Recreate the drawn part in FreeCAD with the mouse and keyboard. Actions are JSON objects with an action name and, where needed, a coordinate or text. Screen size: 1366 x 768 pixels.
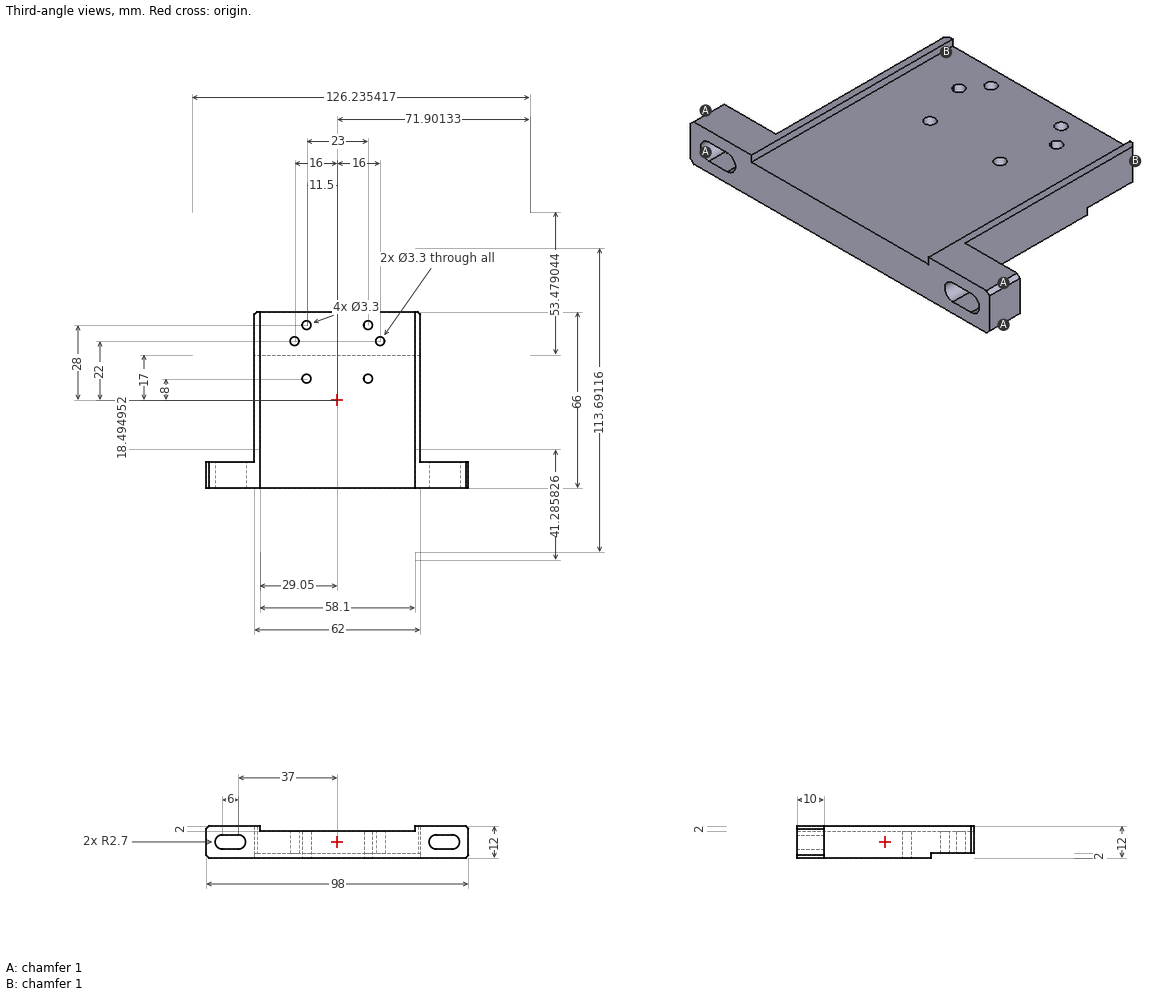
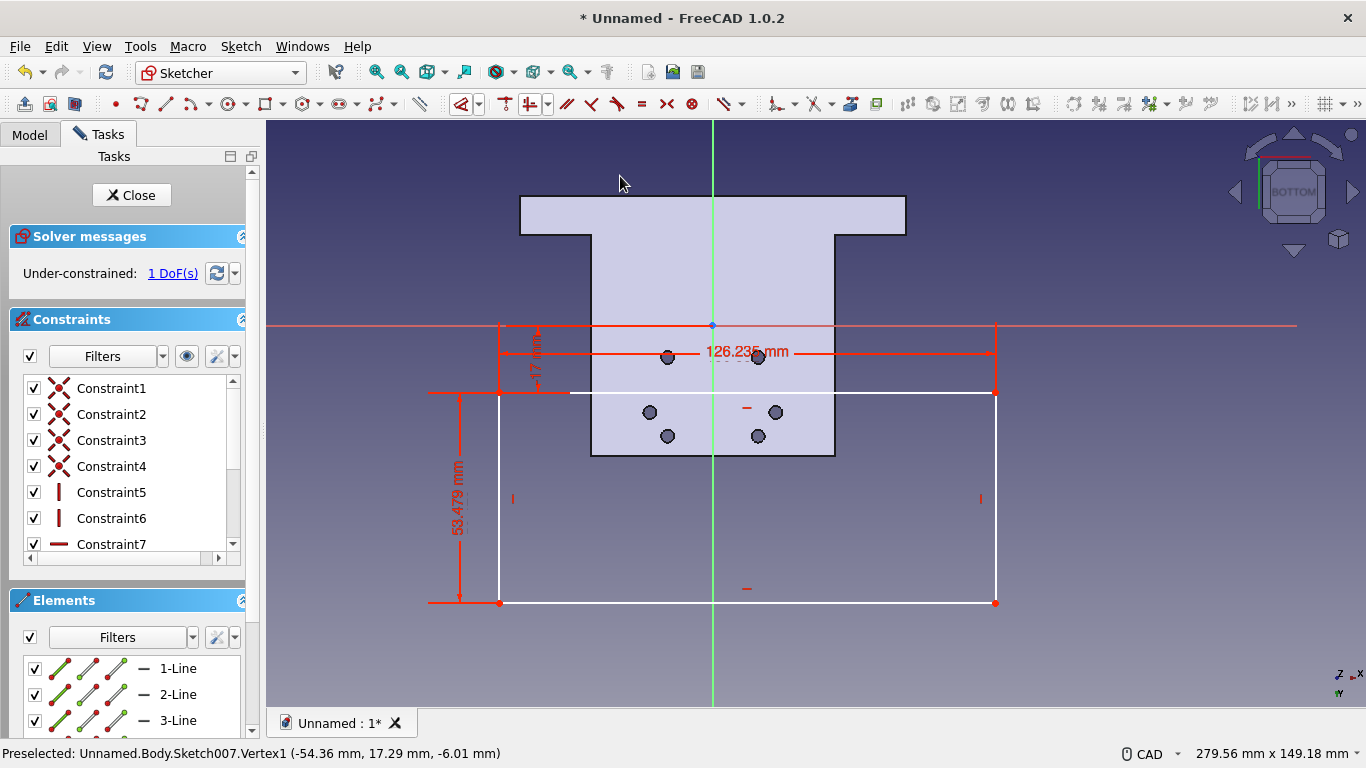
{"action": "left_click", "coordinate": [996, 603]}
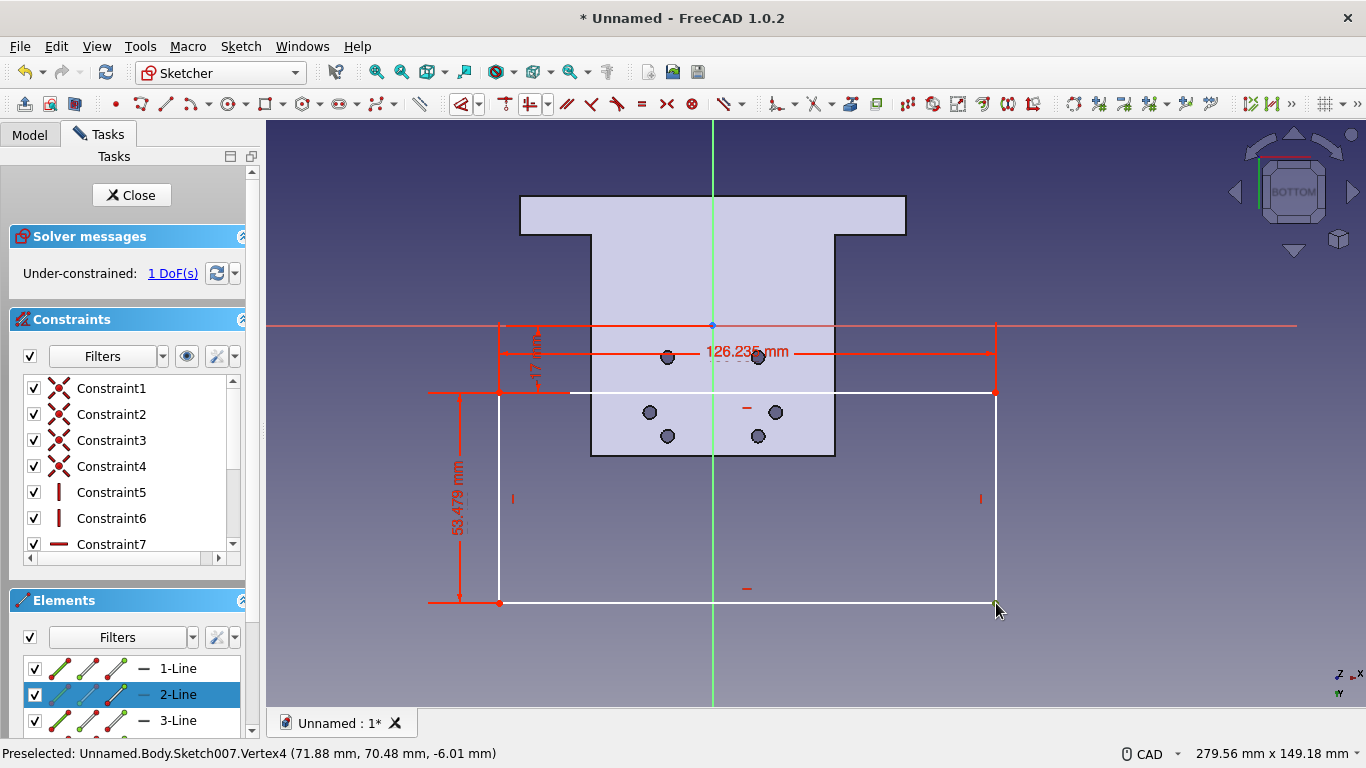
{"action": "left_click", "coordinate": [478, 104]}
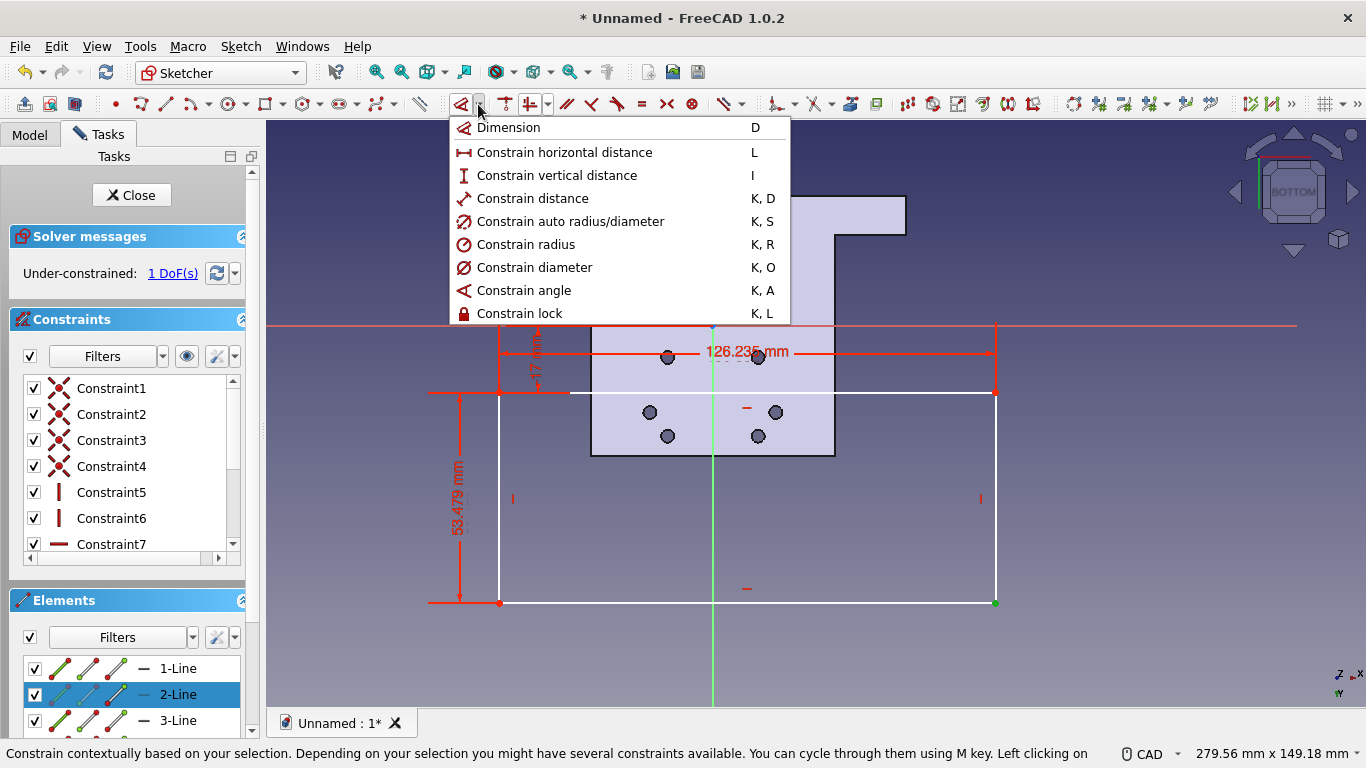
{"action": "left_click", "coordinate": [620, 152]}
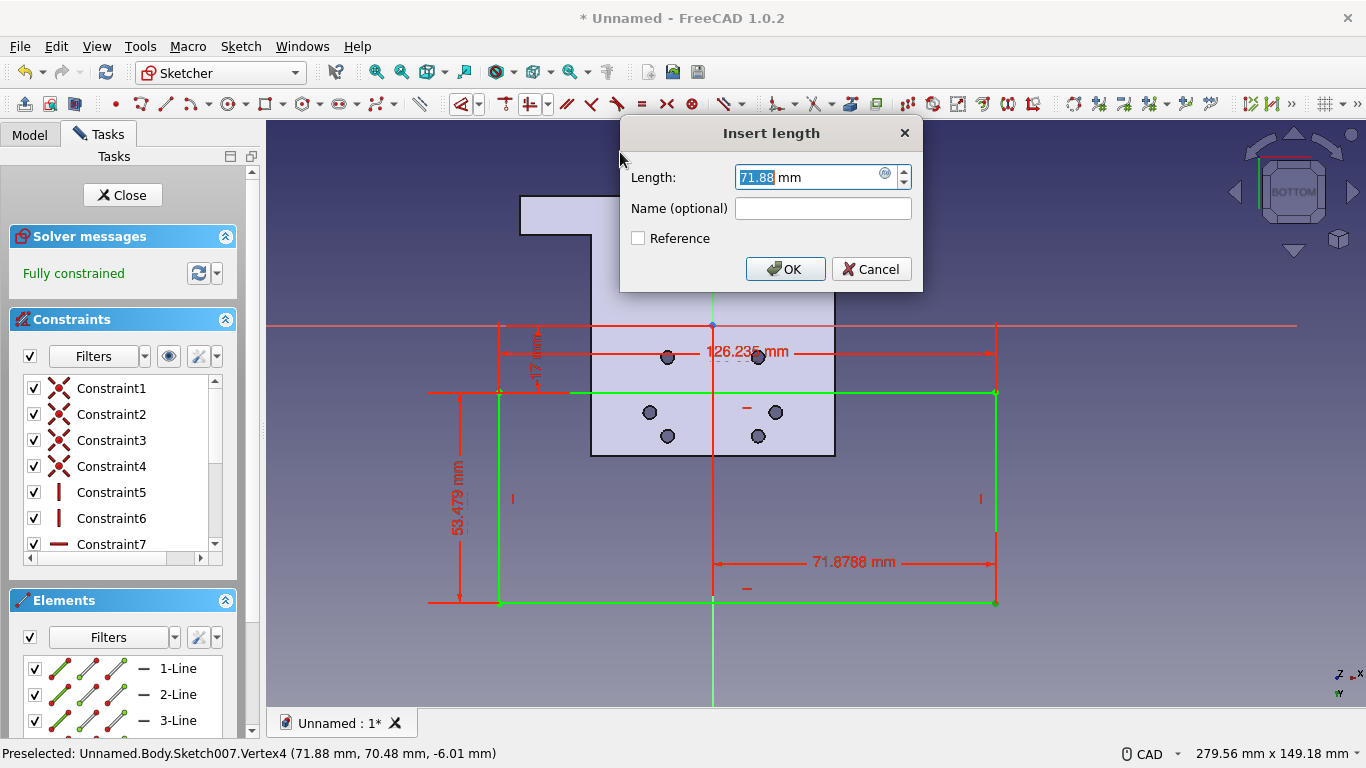
{"action": "type", "text": "71.90133"}
{"action": "key", "text": "Return"}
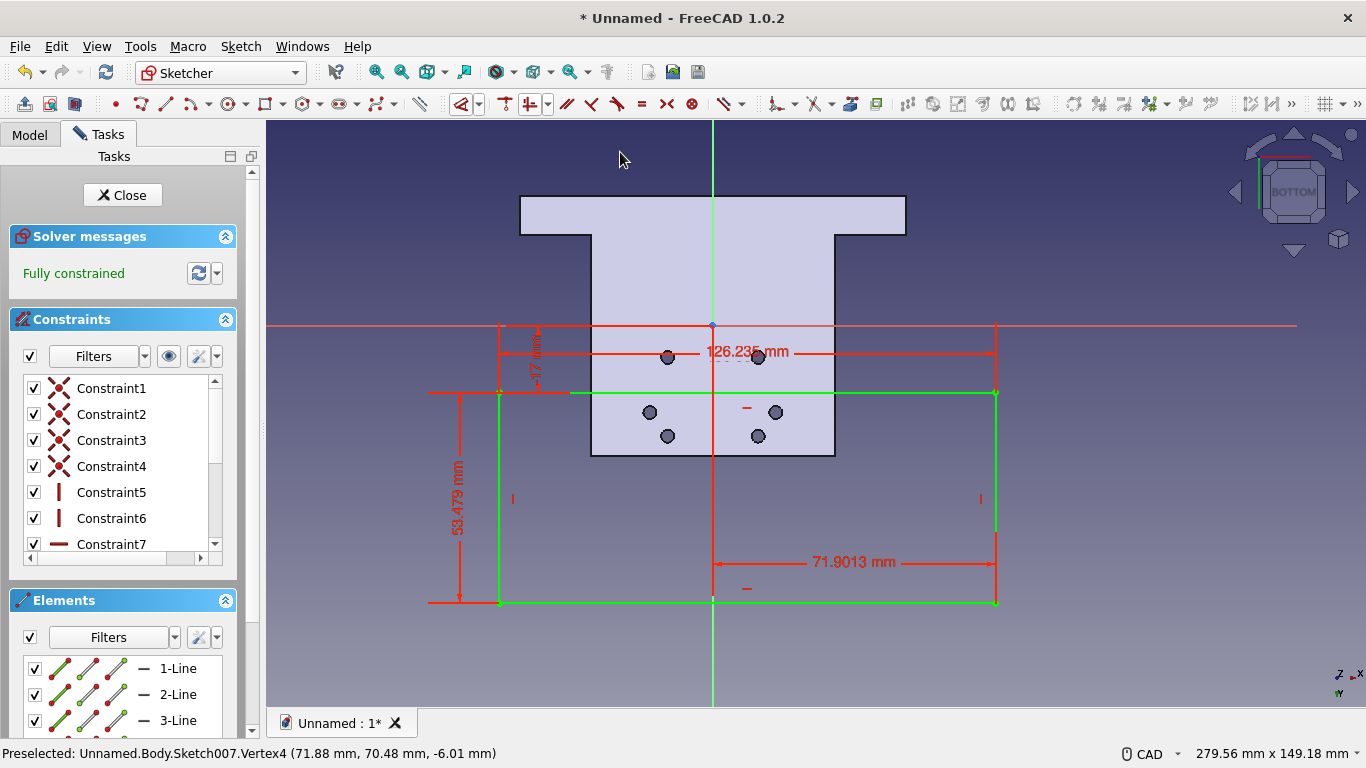
{"action": "left_click", "coordinate": [123, 195]}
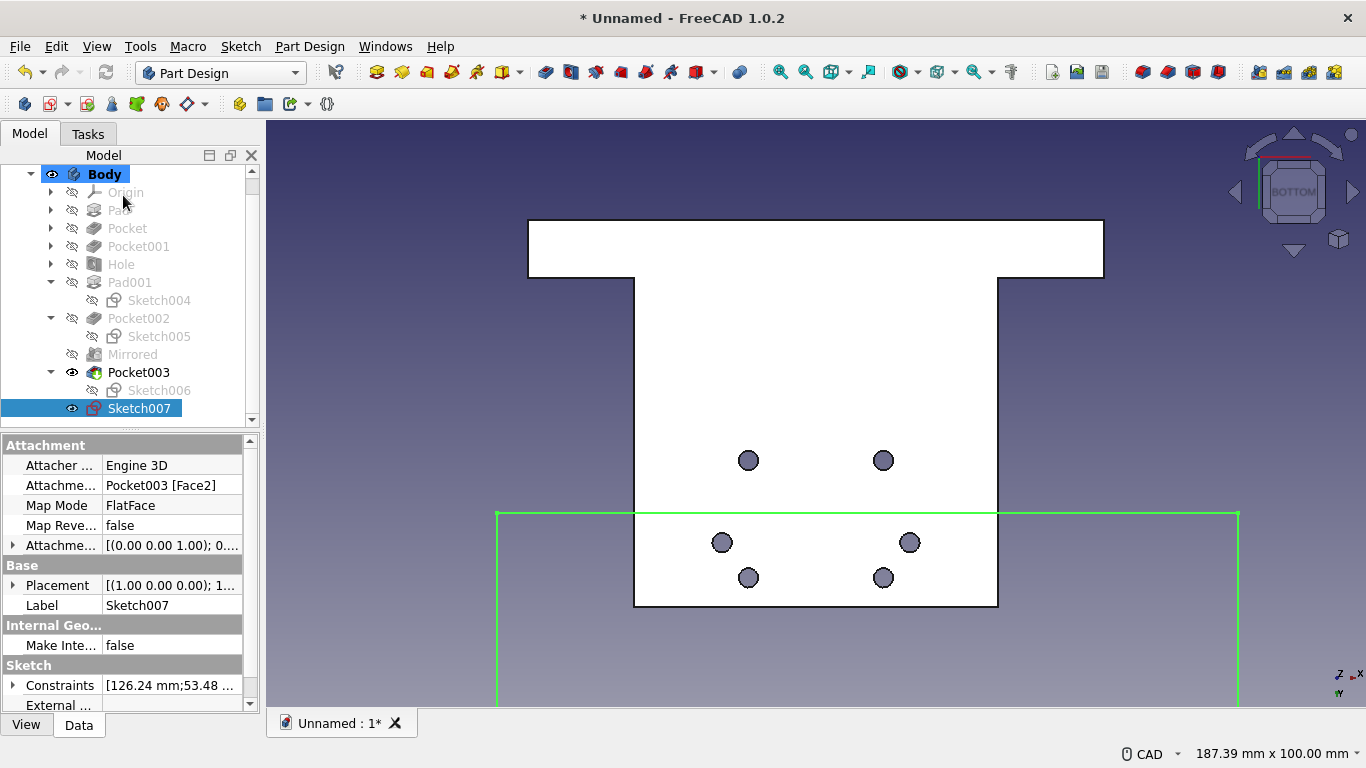
{"action": "left_click", "coordinate": [546, 72]}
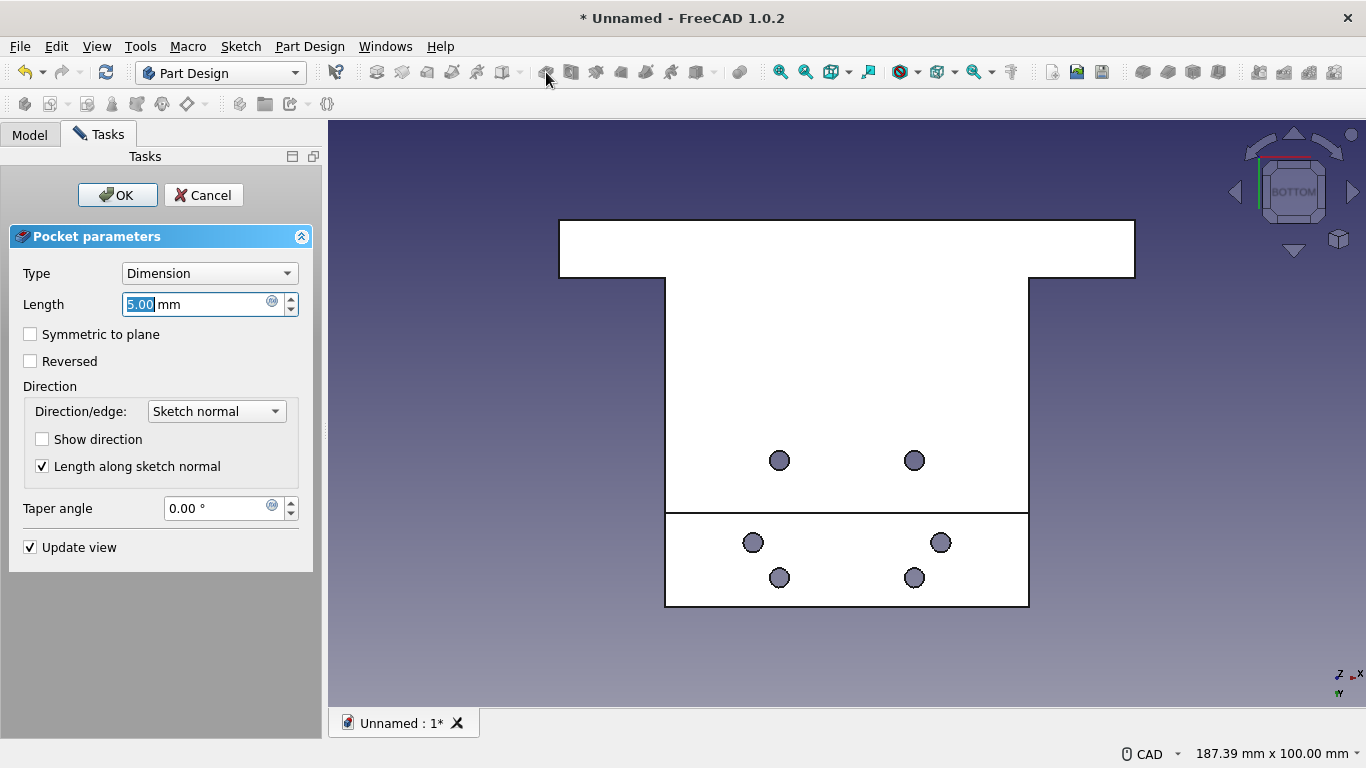
{"action": "type", "text": "2"}
{"action": "key", "text": "Tab"}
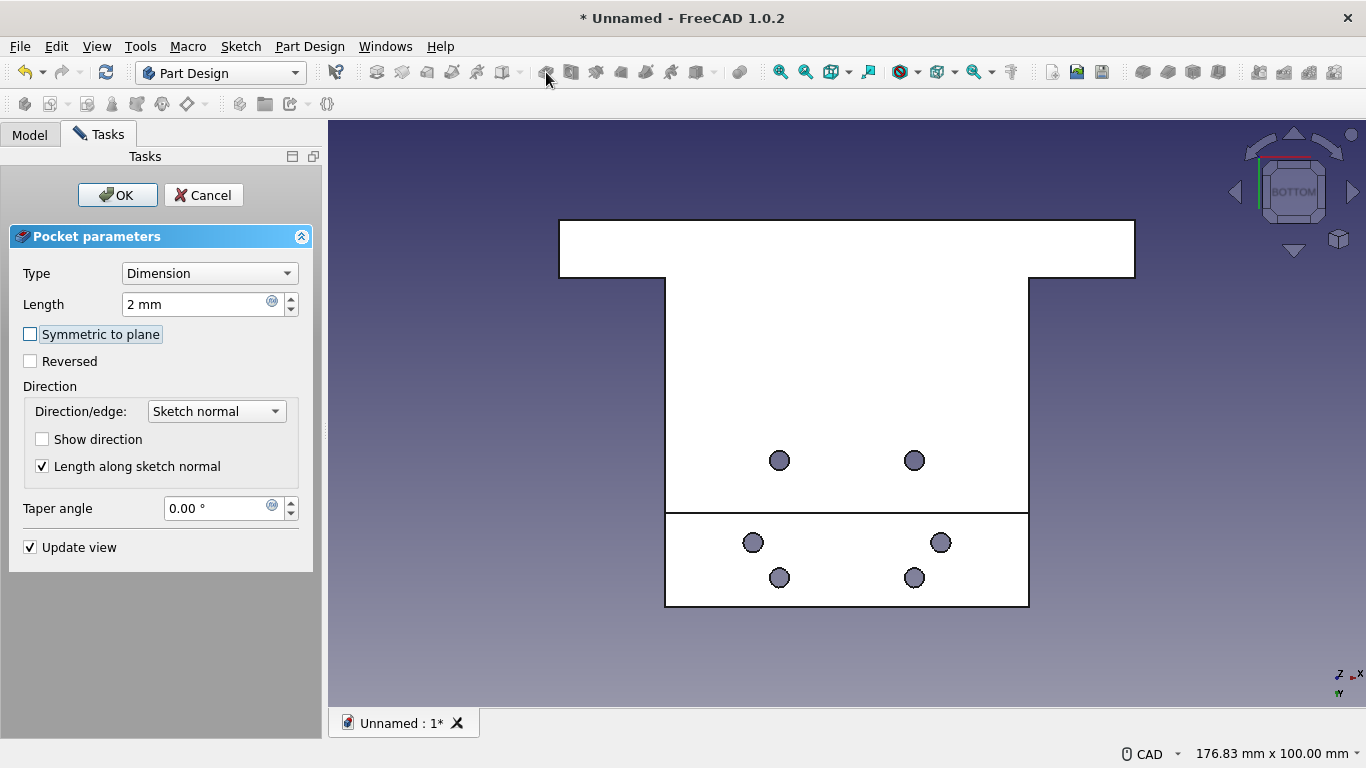
{"action": "left_click", "coordinate": [118, 195]}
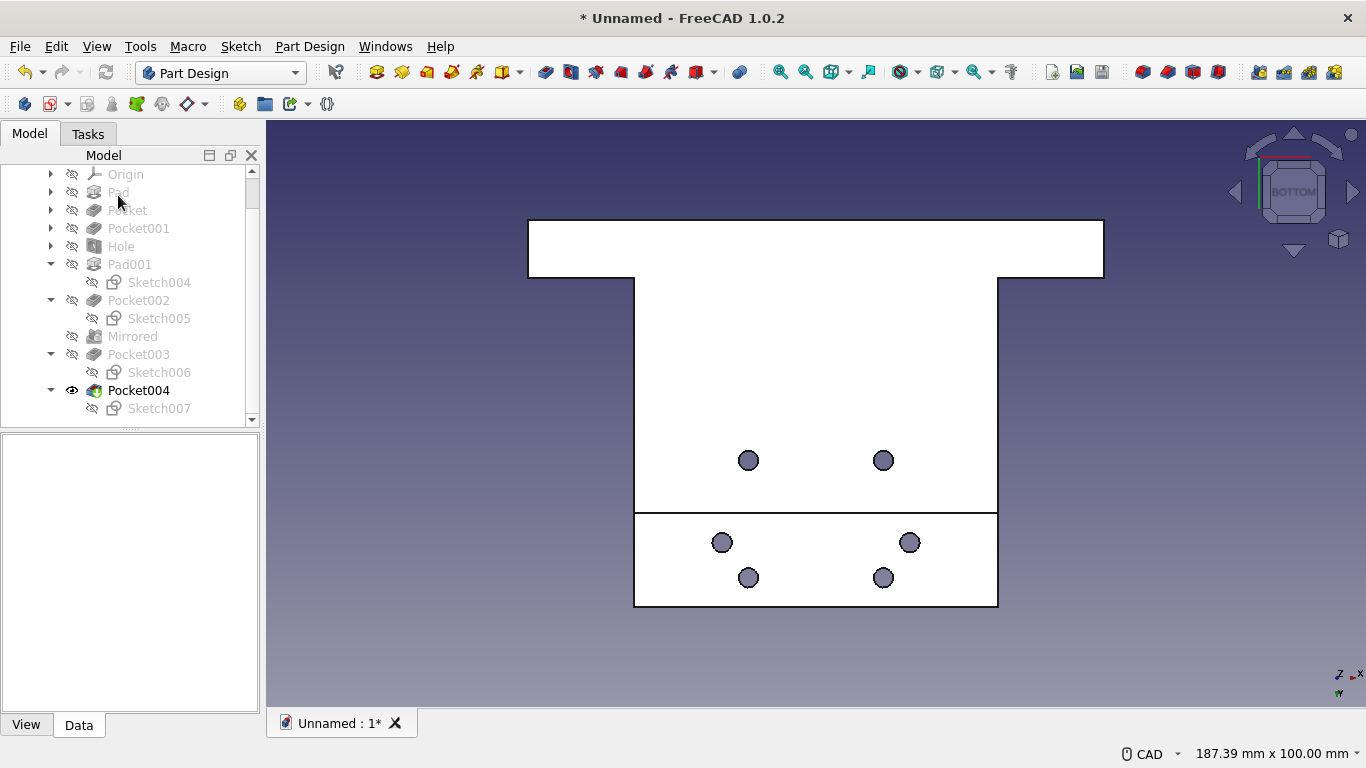
{"action": "left_click", "coordinate": [1104, 248]}